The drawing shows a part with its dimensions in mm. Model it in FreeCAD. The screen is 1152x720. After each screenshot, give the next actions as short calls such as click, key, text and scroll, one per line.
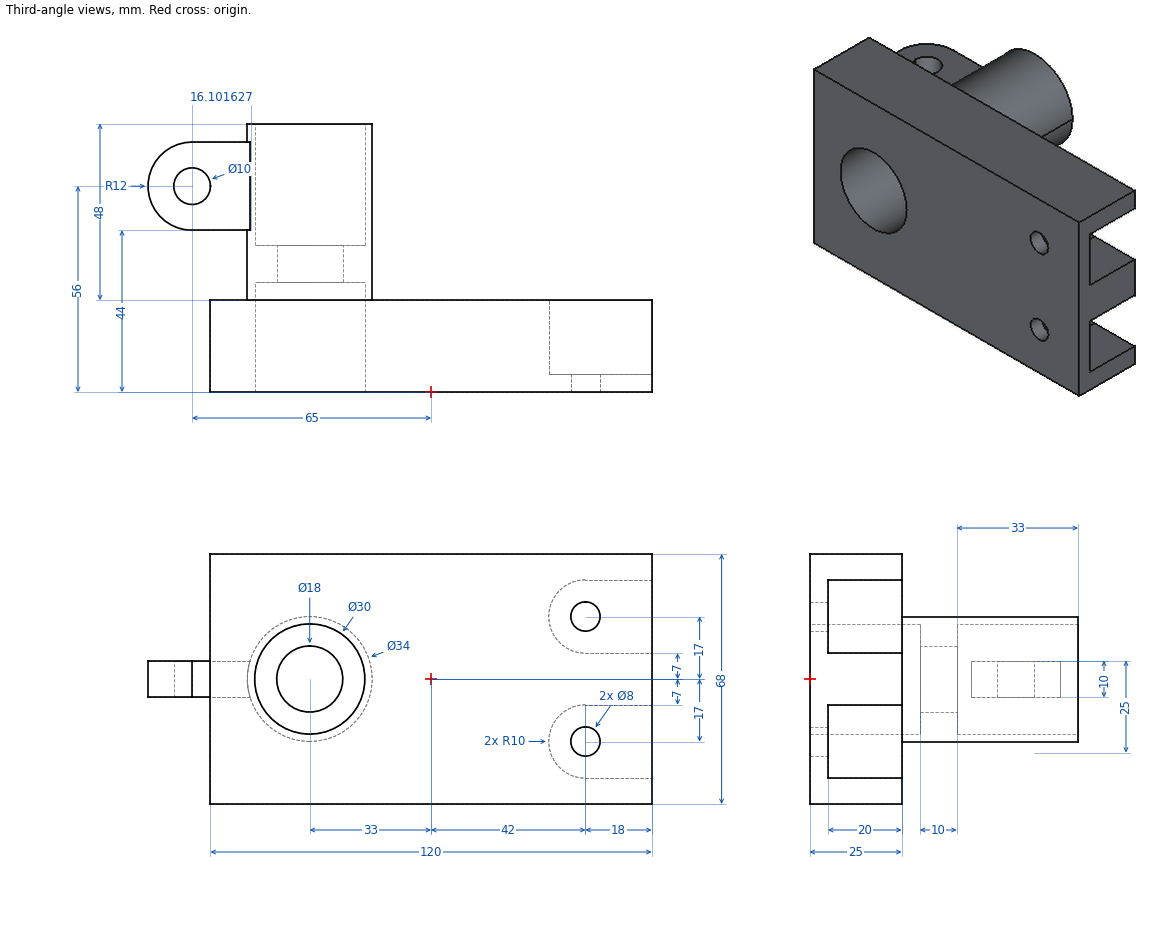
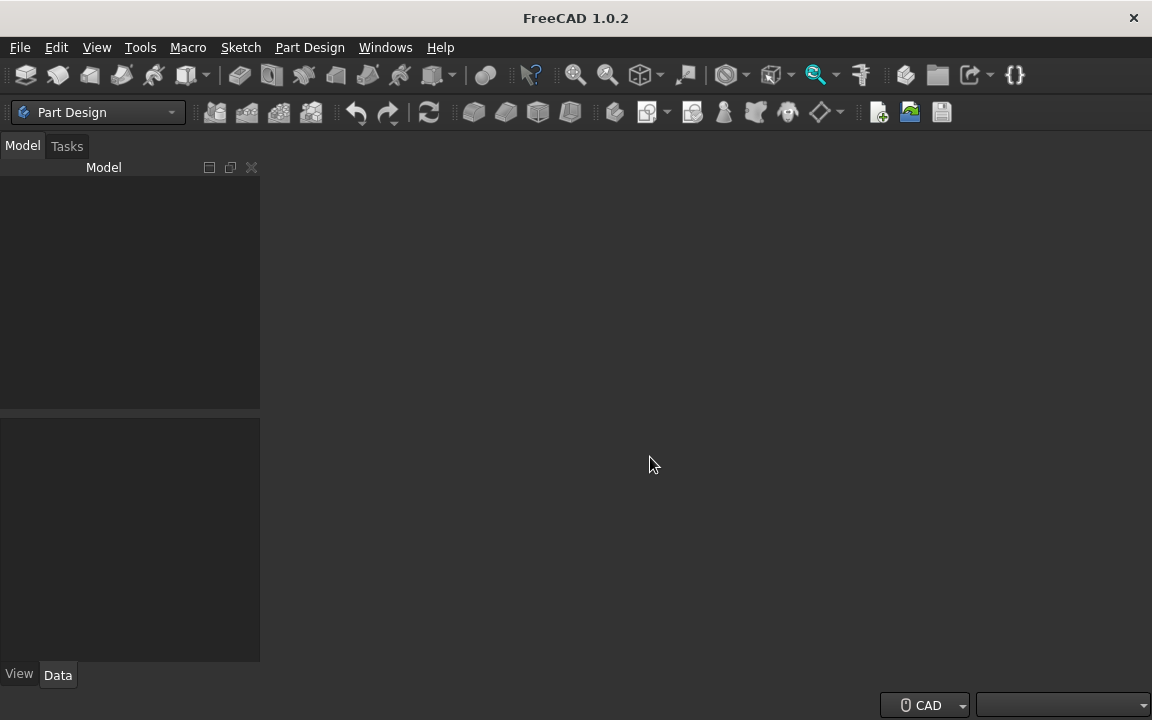
click(878, 112)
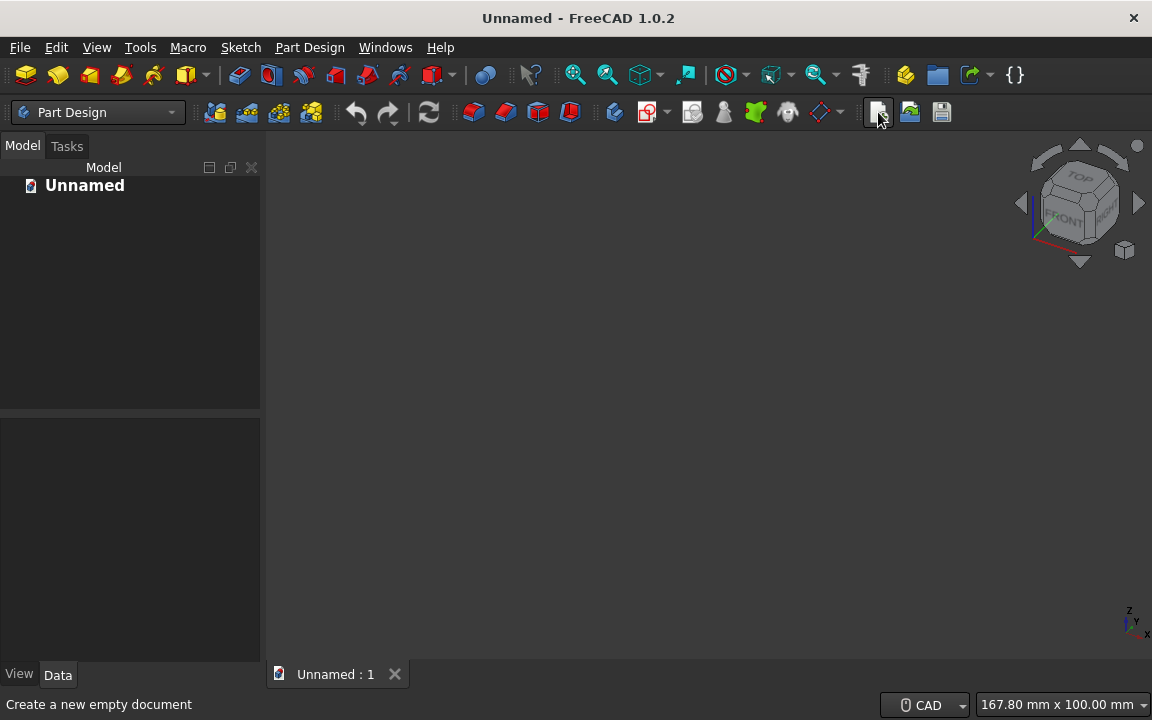
click(648, 112)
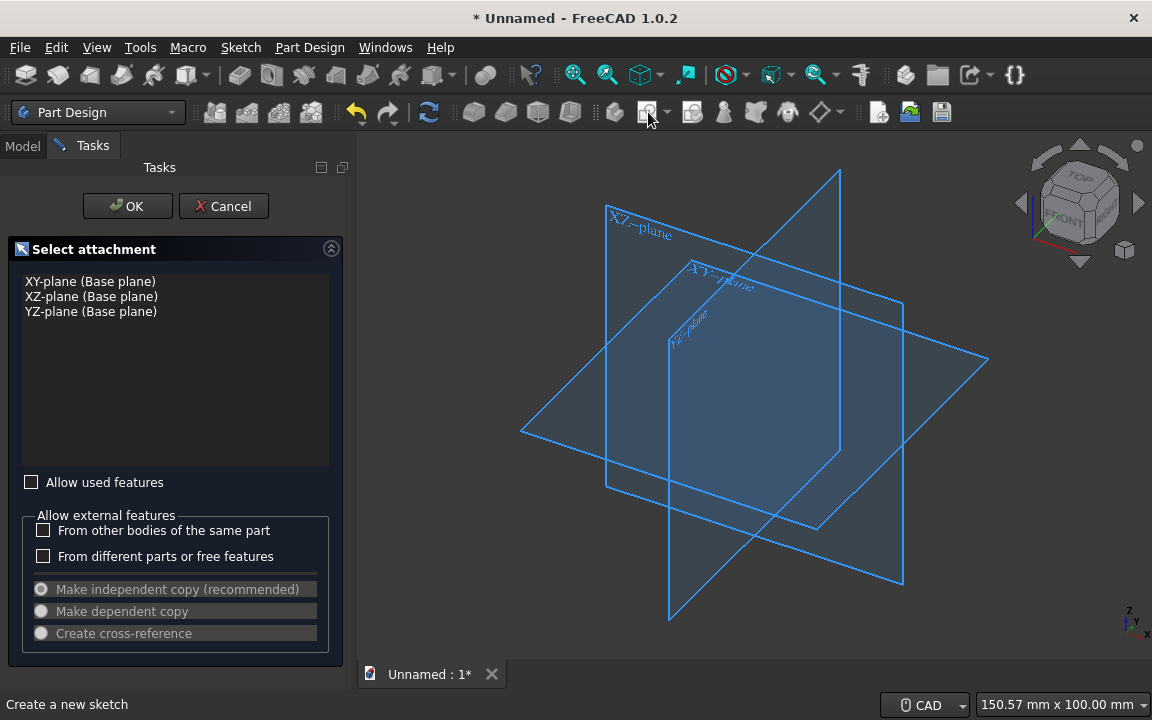
click(82, 296)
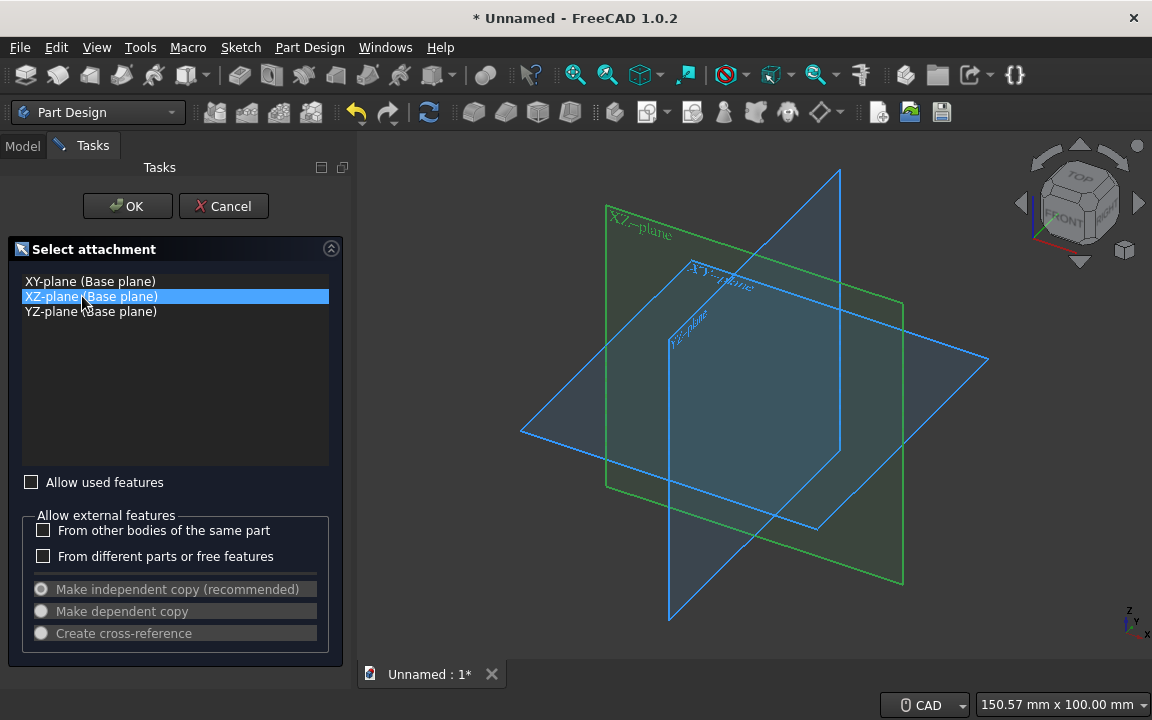
click(128, 206)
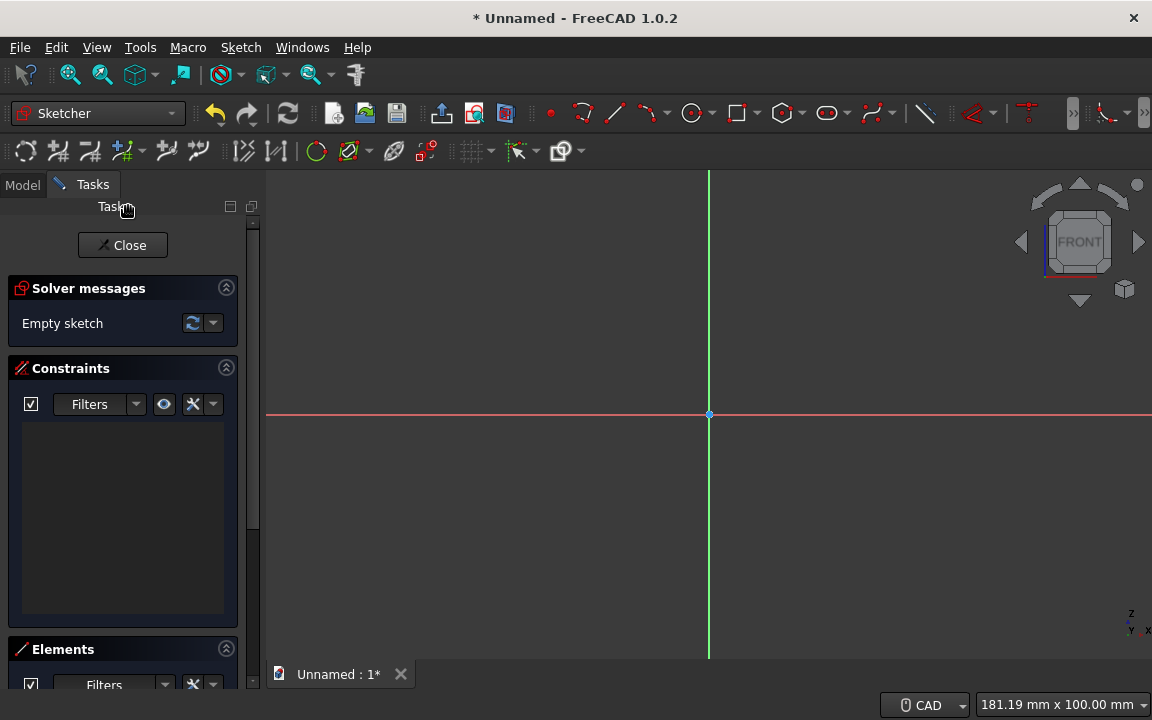
scroll(331, 415, down, 1)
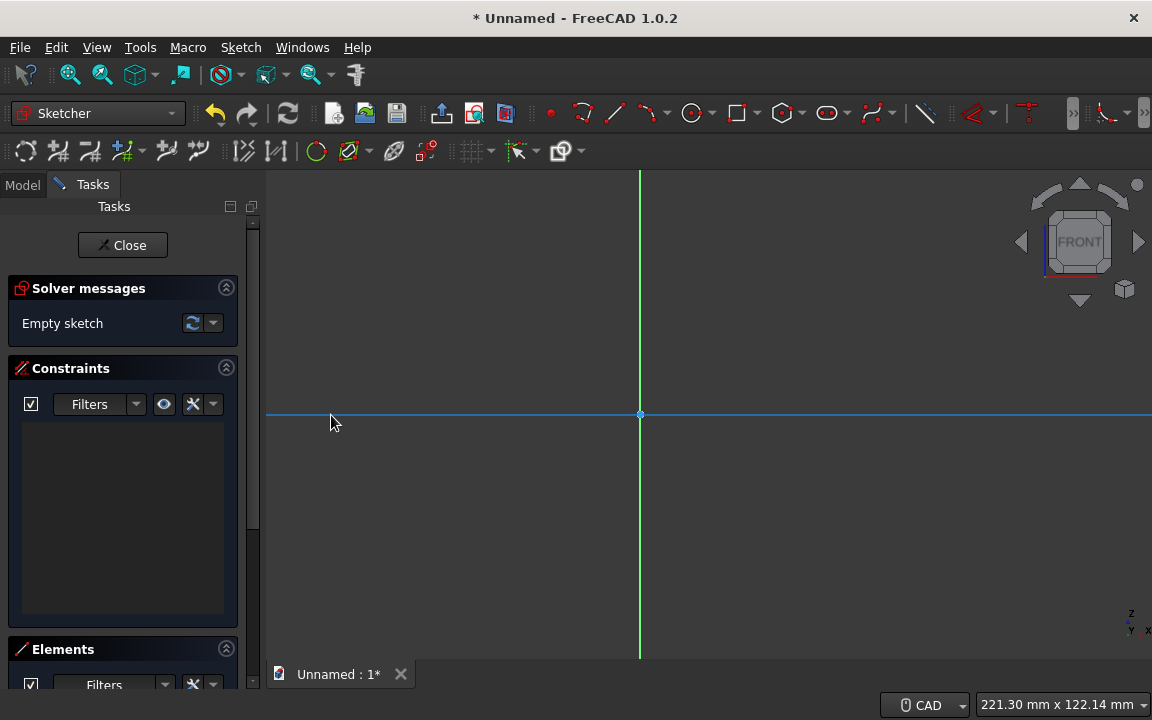
key(g)
key(v)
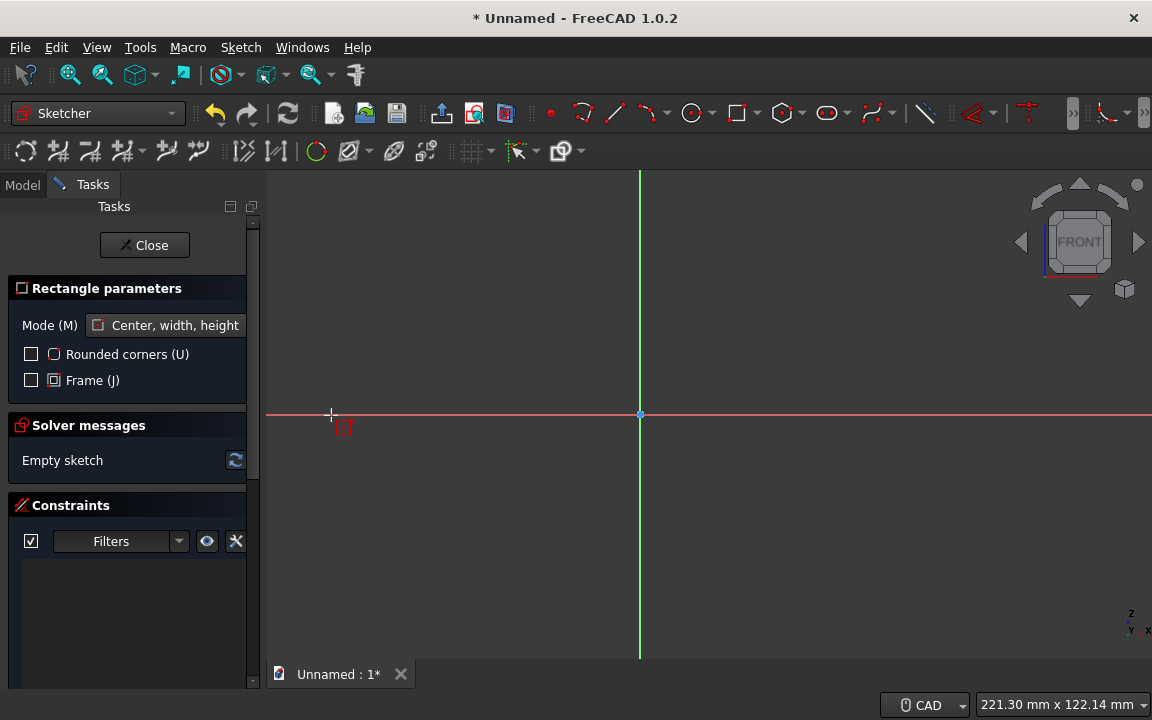
click(640, 415)
move(881, 279)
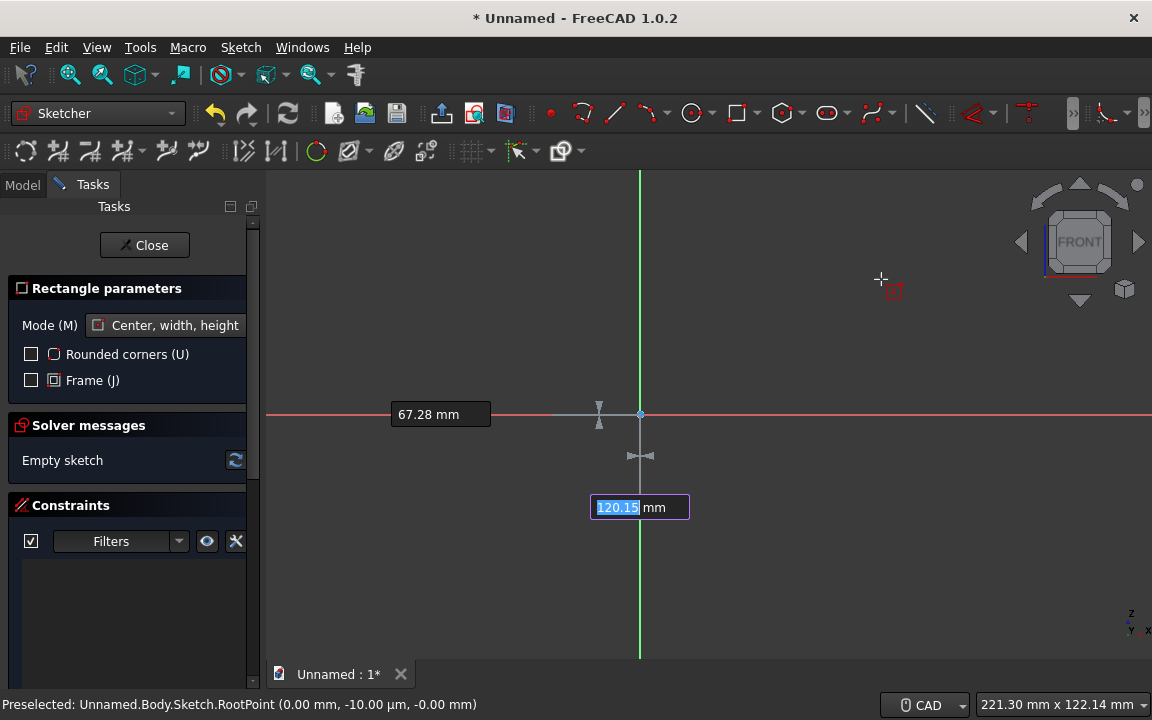
text(120)
key(Tab)
text(68)
key(Return)
key(Escape)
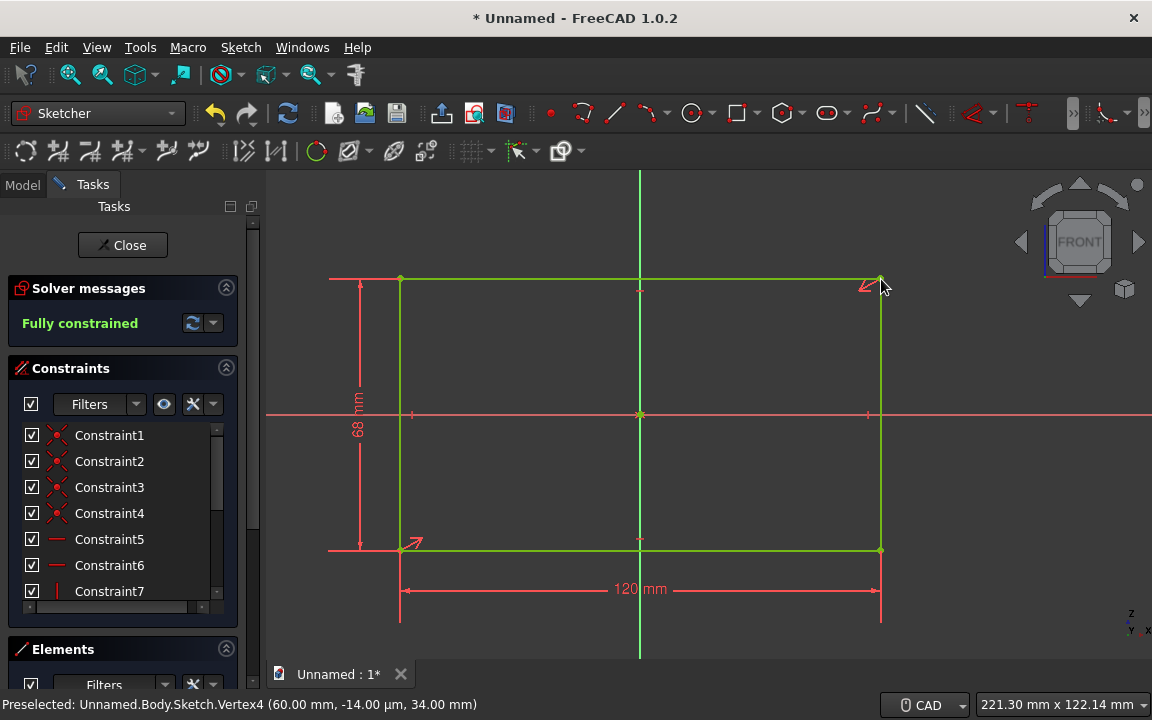
click(123, 245)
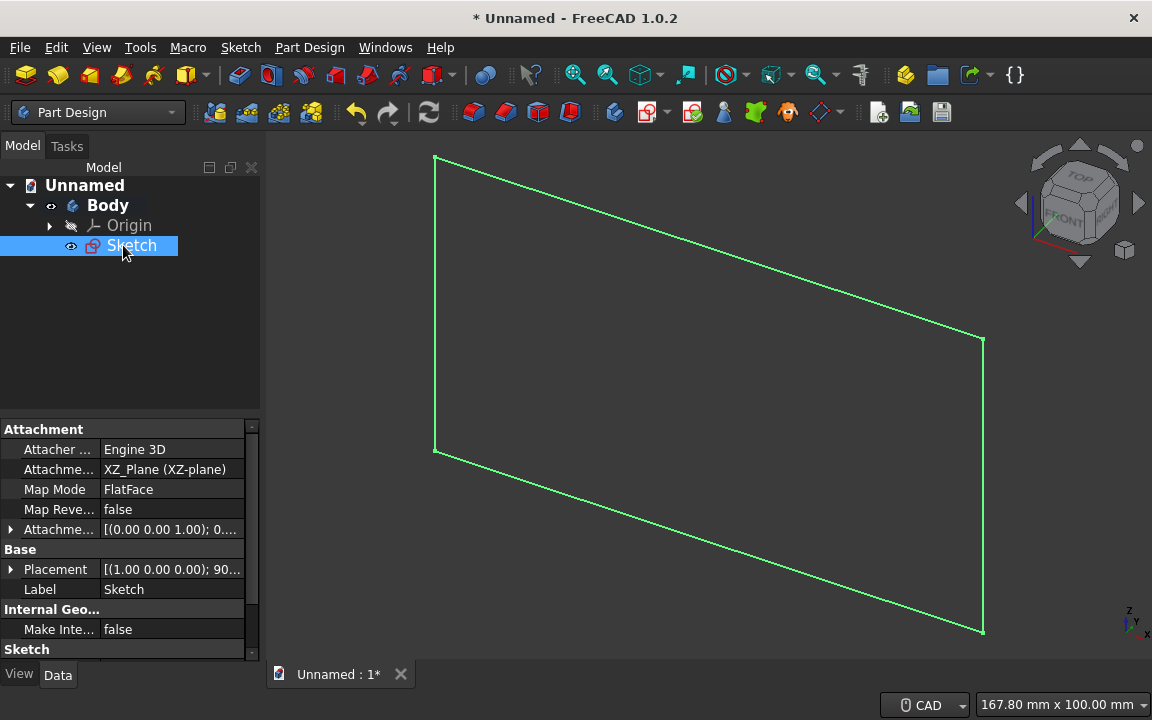
click(26, 76)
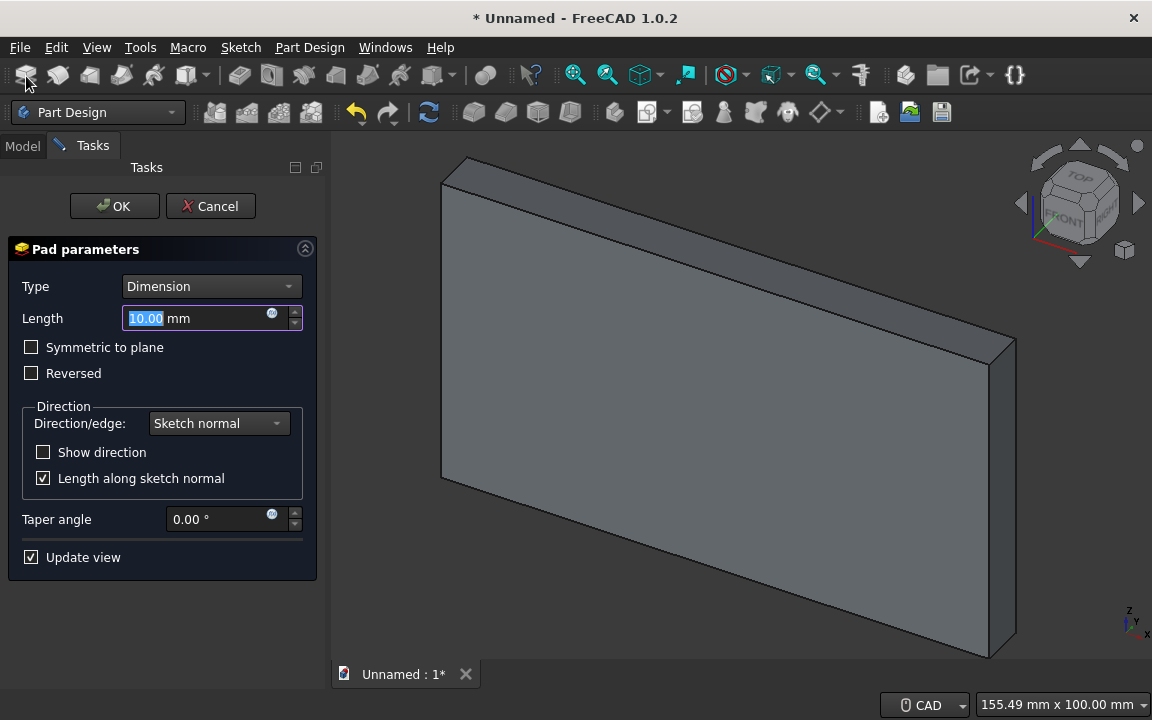
text(25)
key(Tab)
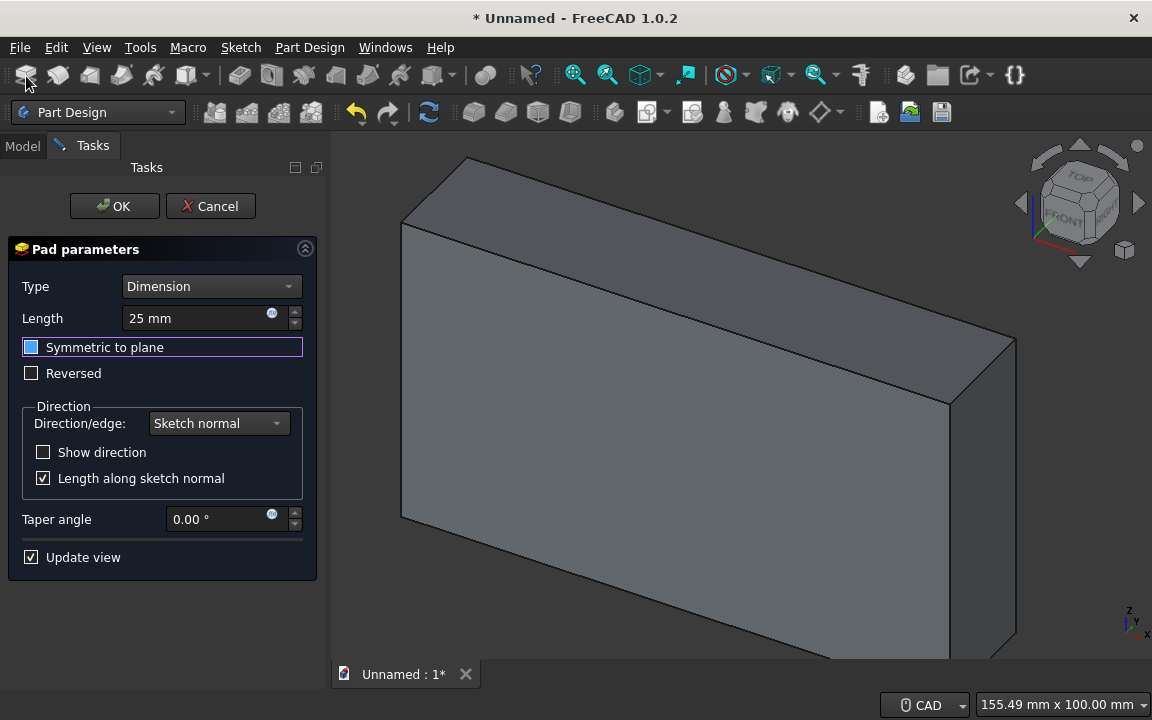
click(30, 373)